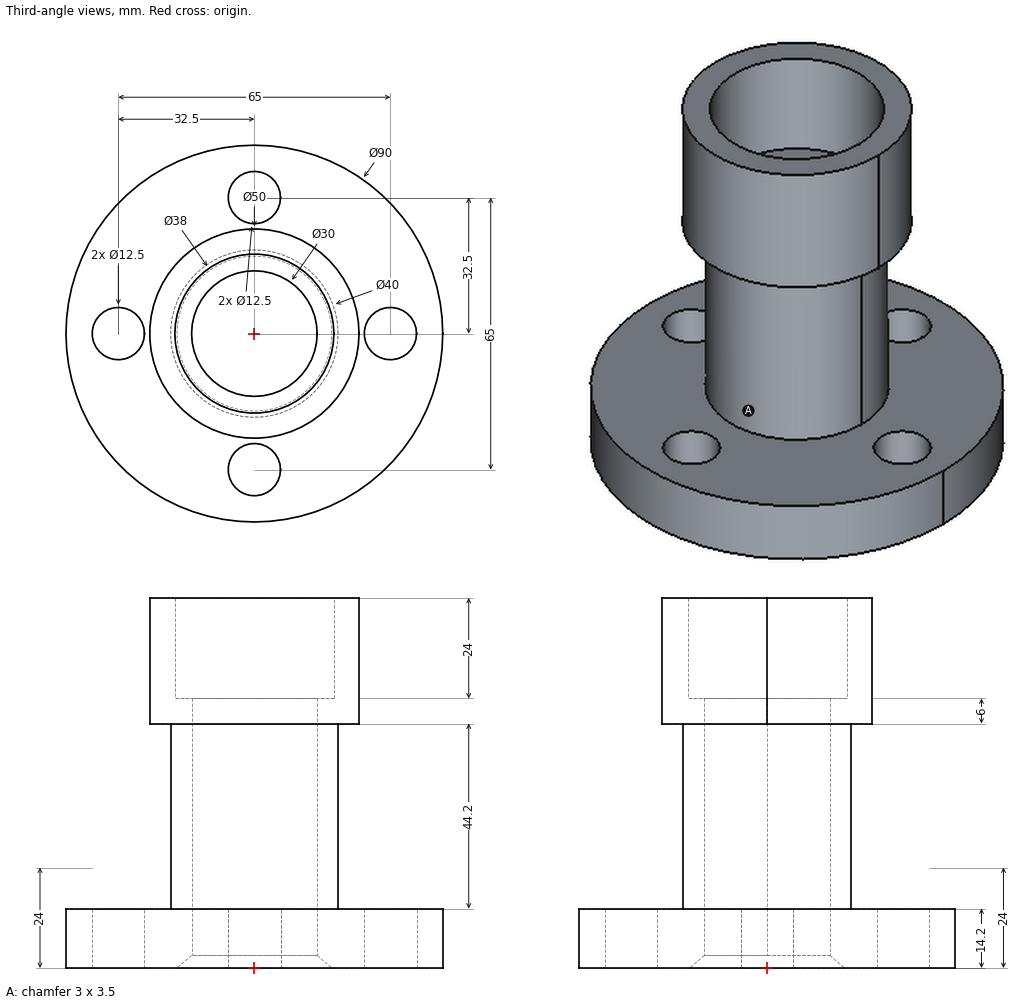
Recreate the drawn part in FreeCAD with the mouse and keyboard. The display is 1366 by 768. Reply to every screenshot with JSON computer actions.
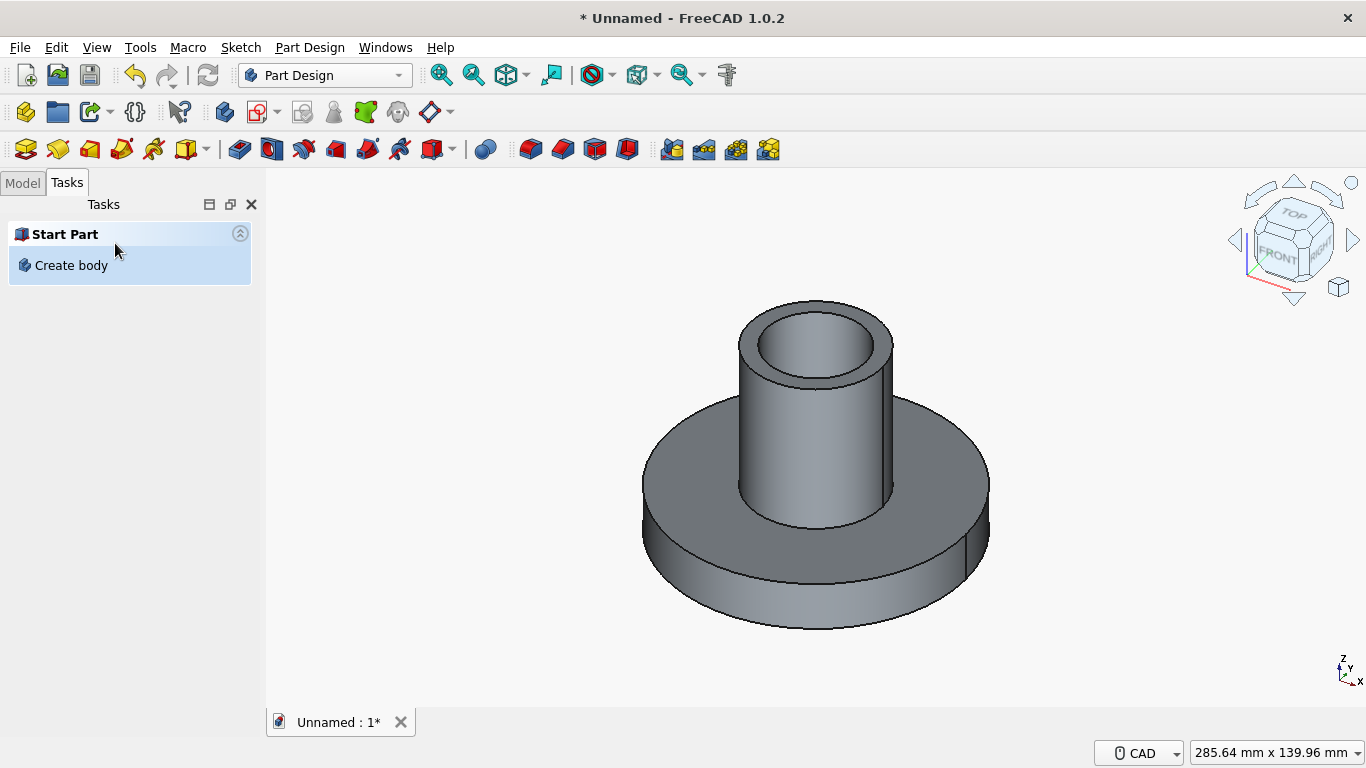
{"action": "left_click", "coordinate": [748, 336]}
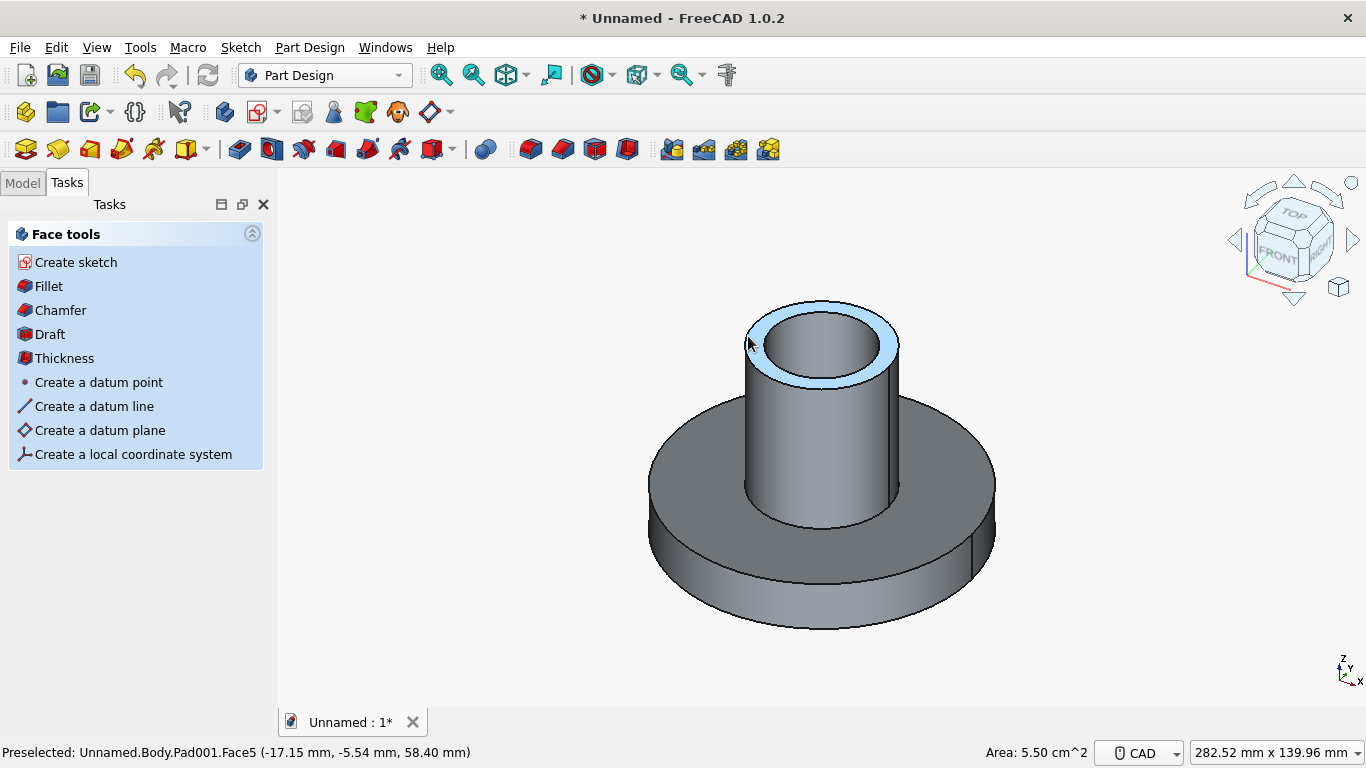
{"action": "left_click", "coordinate": [258, 112]}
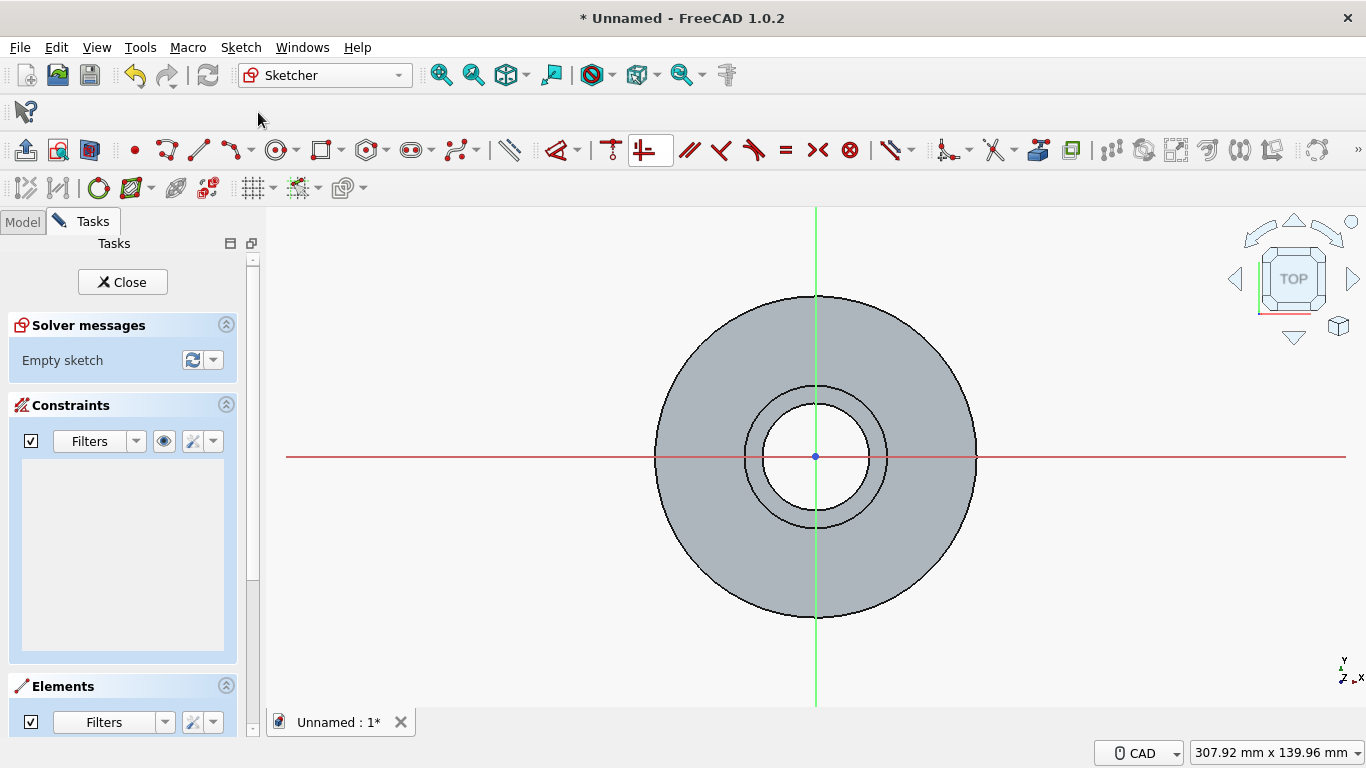
{"action": "scroll", "coordinate": [899, 457], "scroll_direction": "up", "scroll_amount": 3}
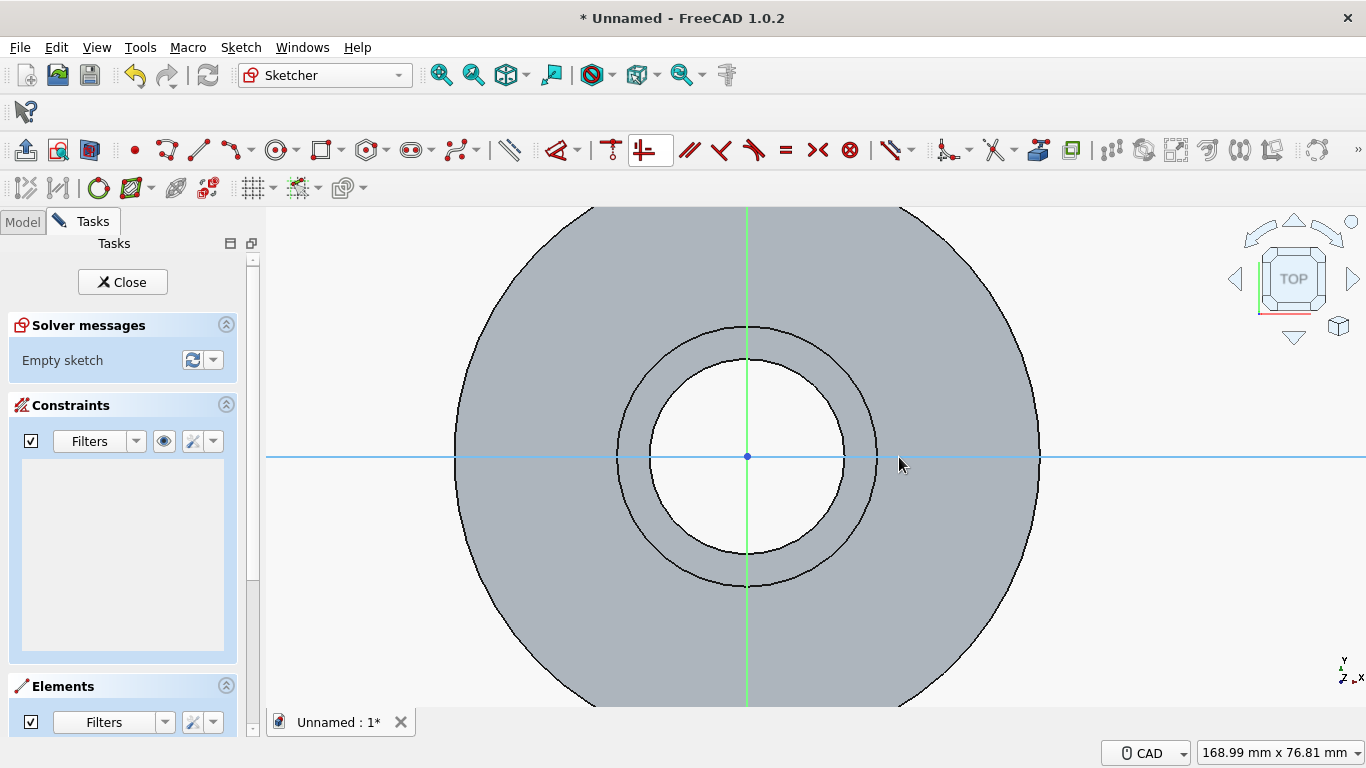
{"action": "left_click", "coordinate": [276, 150]}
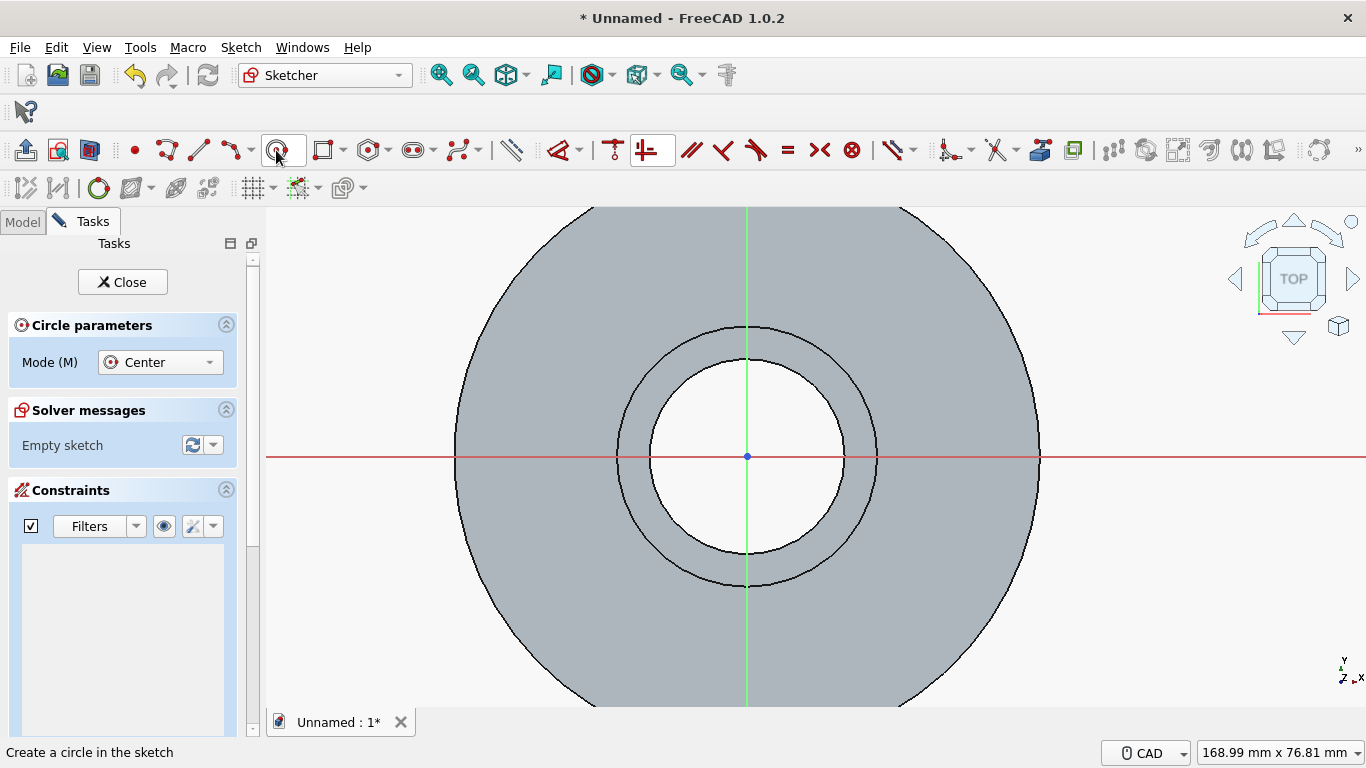
{"action": "left_click", "coordinate": [747, 457]}
{"action": "mouse_move", "coordinate": [862, 342]}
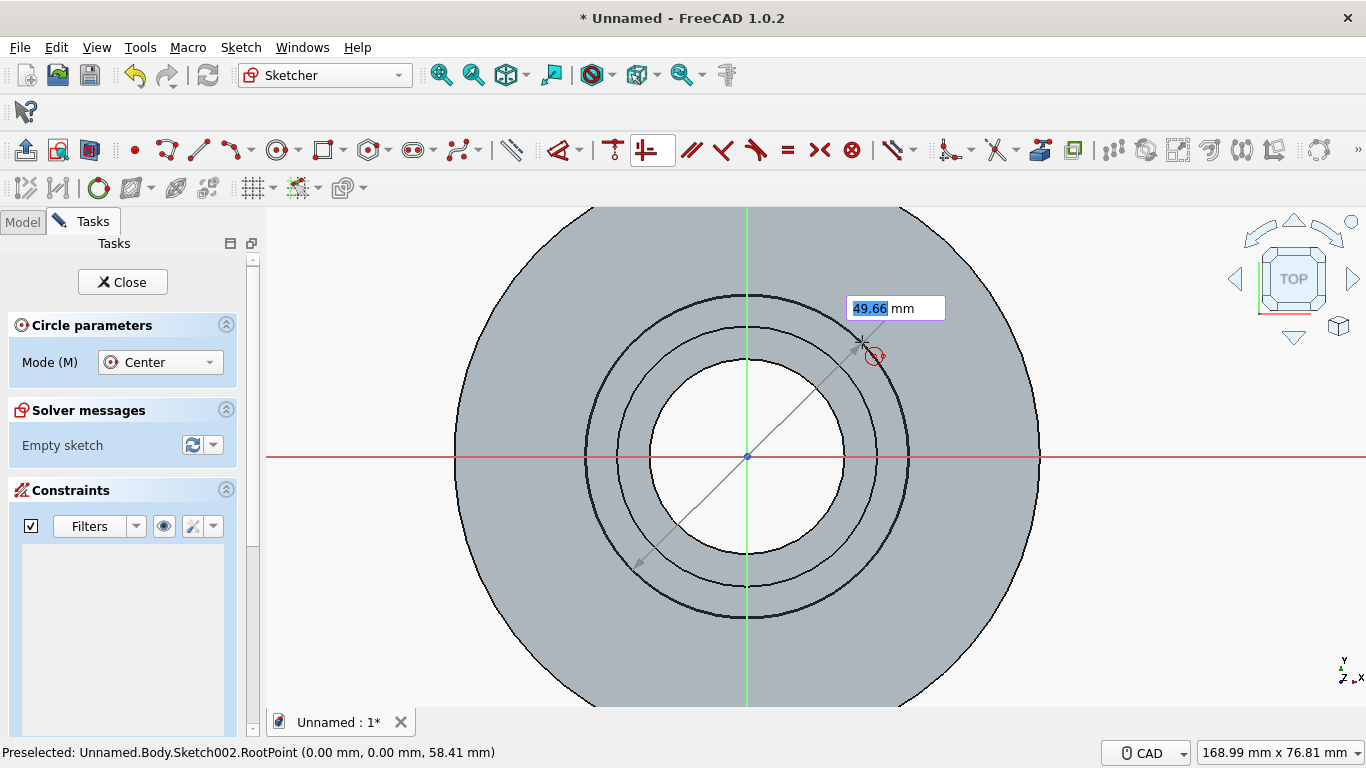
{"action": "type", "text": "50"}
{"action": "key", "text": "Return"}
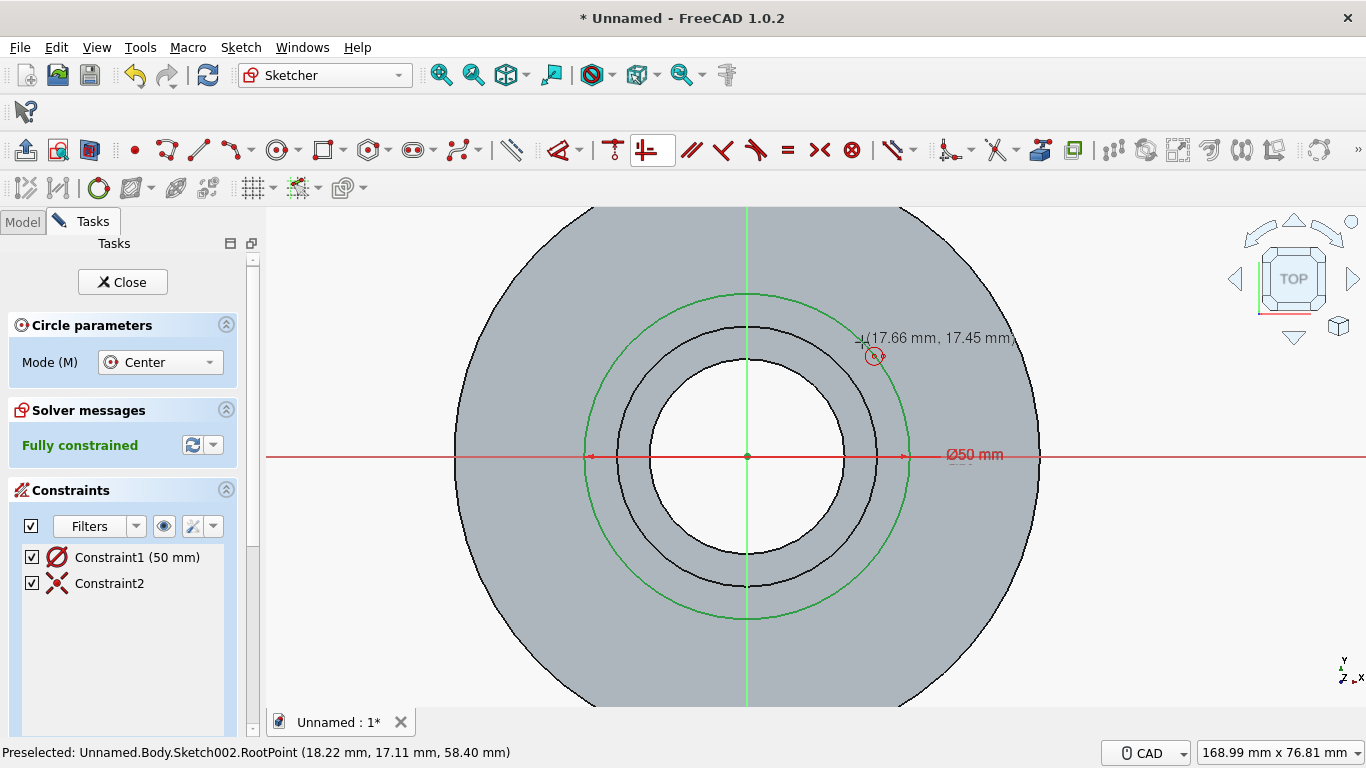
{"action": "left_click", "coordinate": [747, 457]}
{"action": "mouse_move", "coordinate": [816, 388]}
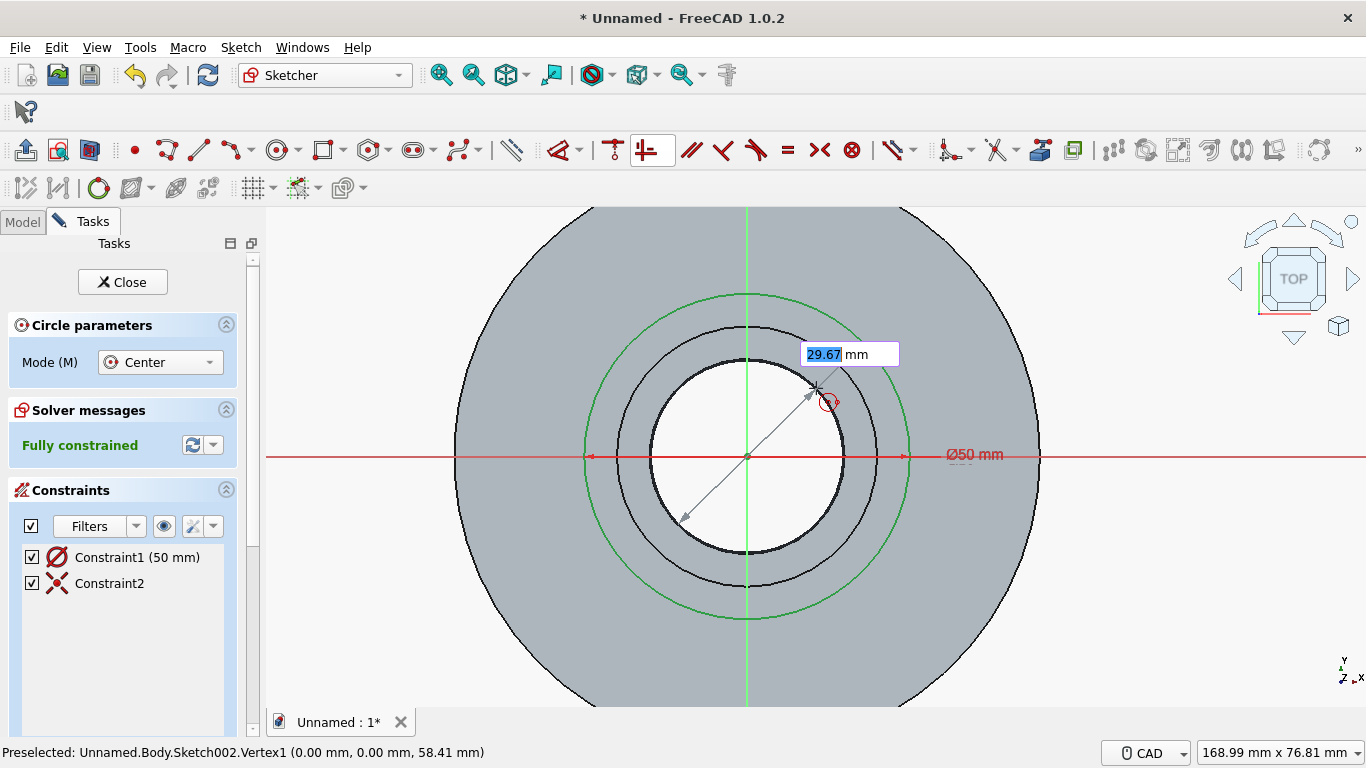
{"action": "type", "text": "30"}
{"action": "key", "text": "Return"}
{"action": "key", "text": "Escape"}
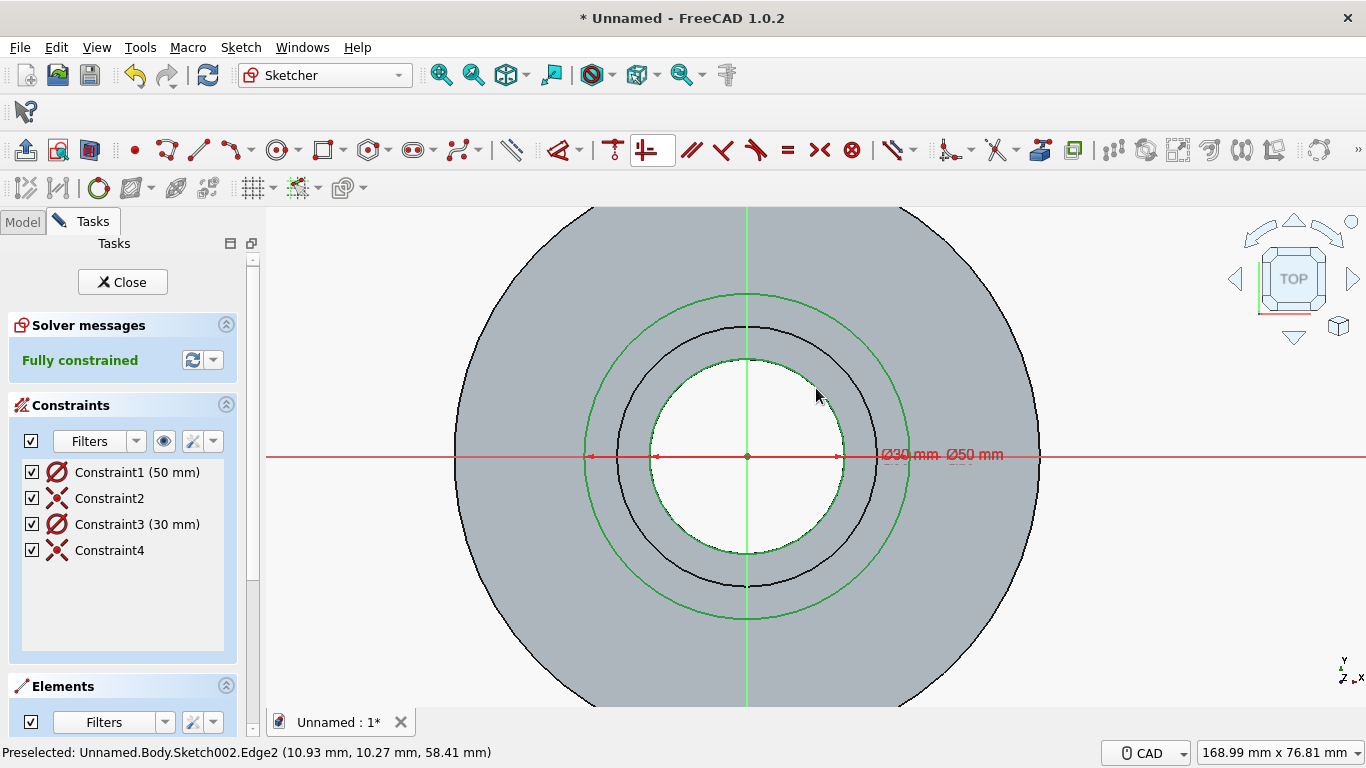
{"action": "left_click", "coordinate": [123, 282]}